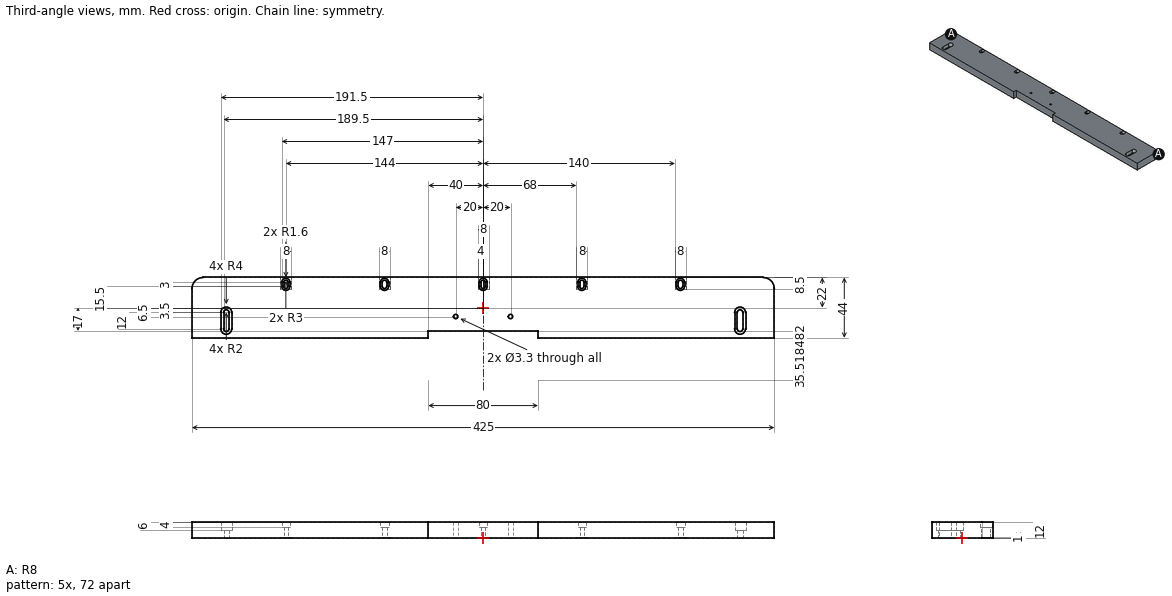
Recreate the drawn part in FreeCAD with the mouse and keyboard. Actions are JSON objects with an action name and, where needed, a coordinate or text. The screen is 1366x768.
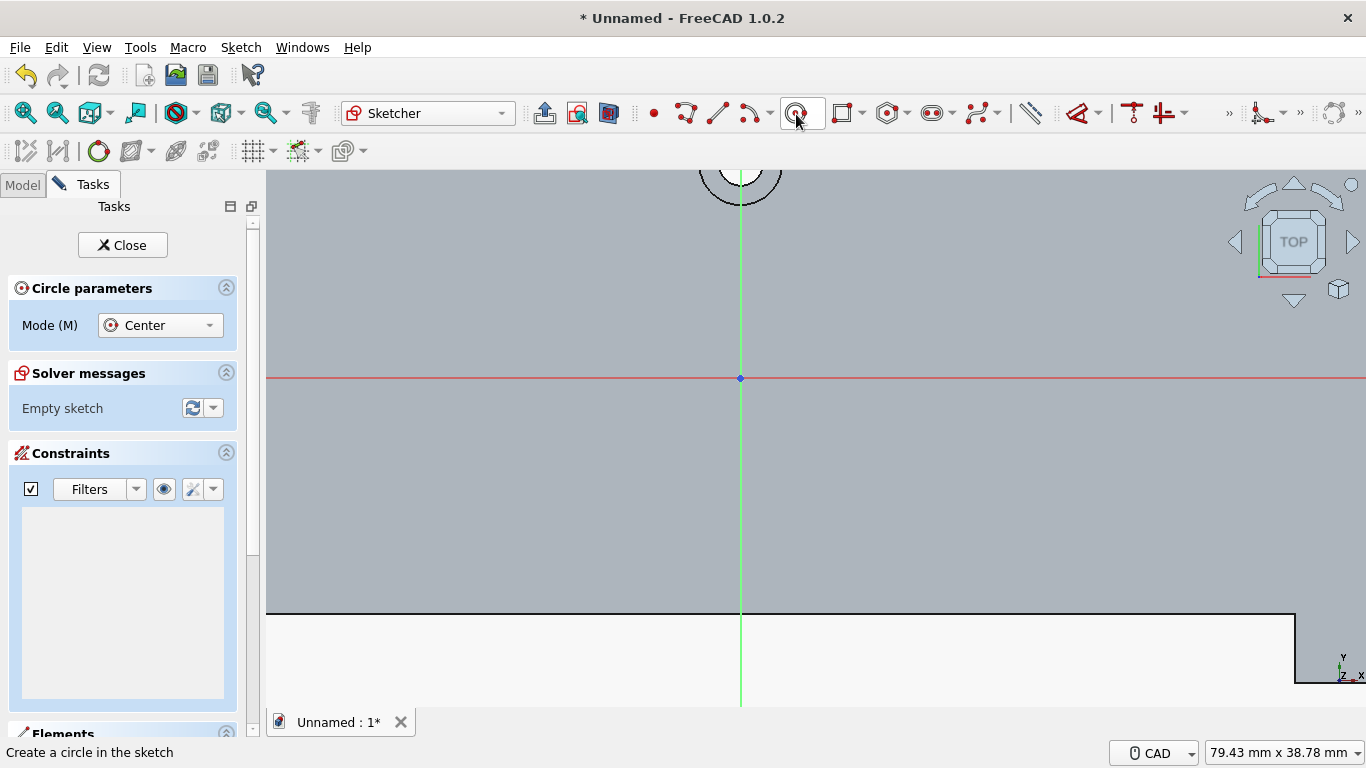
{"action": "left_click", "coordinate": [464, 468]}
{"action": "mouse_move", "coordinate": [480, 452]}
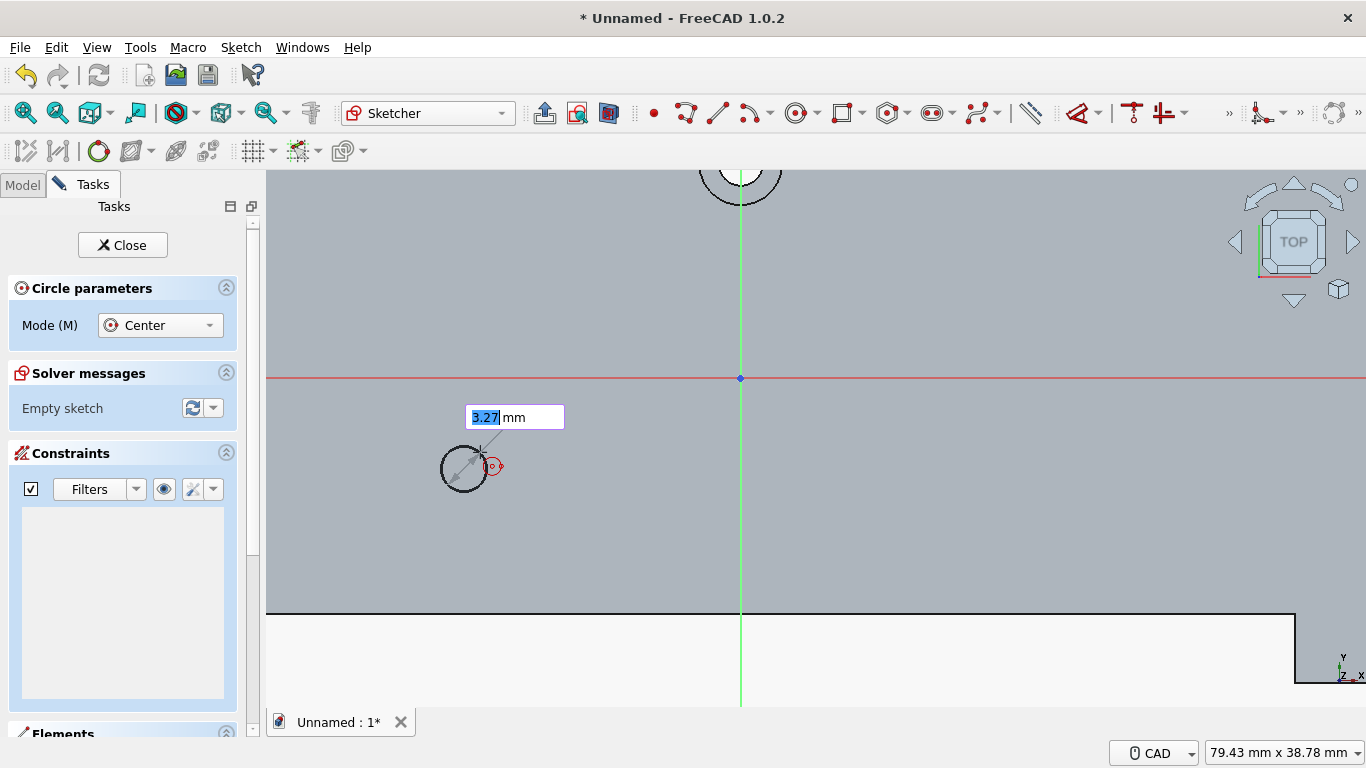
{"action": "type", "text": "3.3"}
{"action": "key", "text": "Return"}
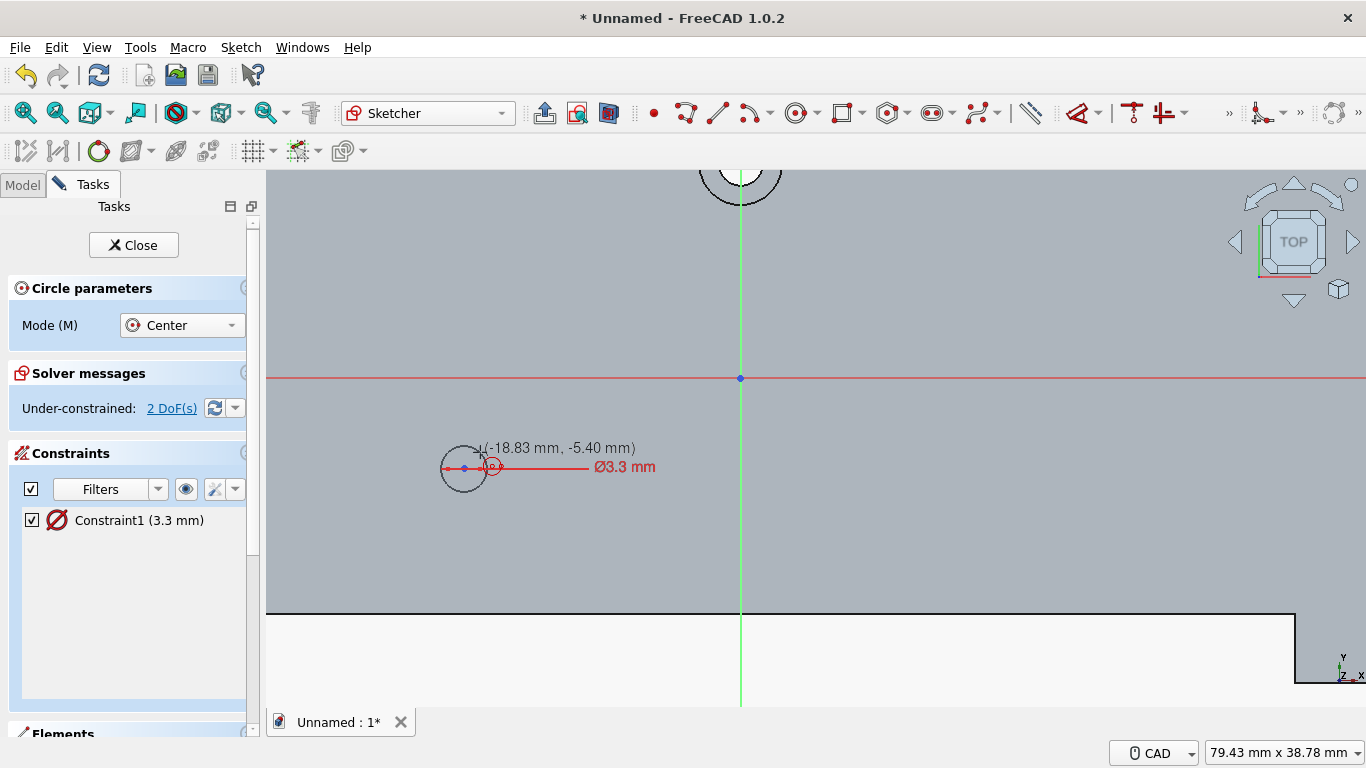
{"action": "left_click", "coordinate": [1018, 468]}
{"action": "mouse_move", "coordinate": [1034, 452]}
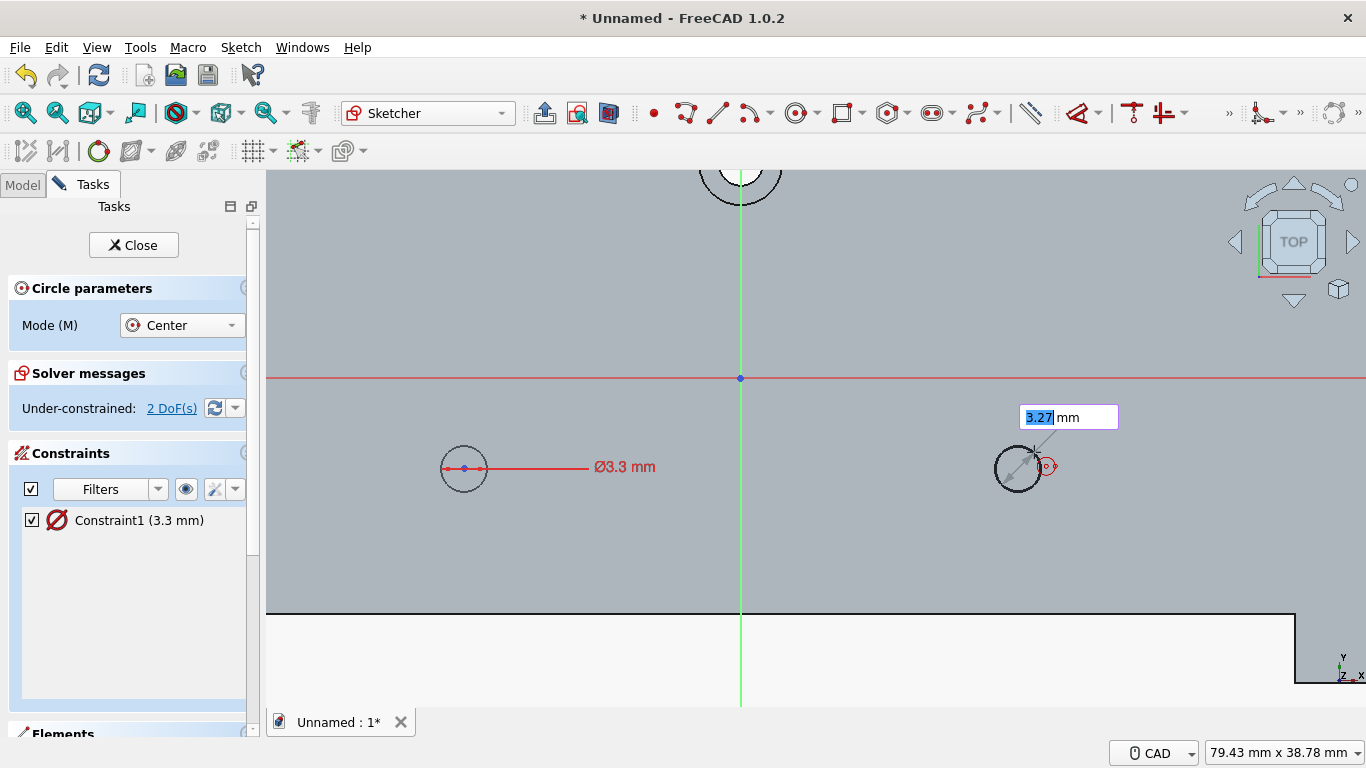
{"action": "type", "text": "3.3"}
{"action": "key", "text": "Return"}
{"action": "key", "text": "Escape"}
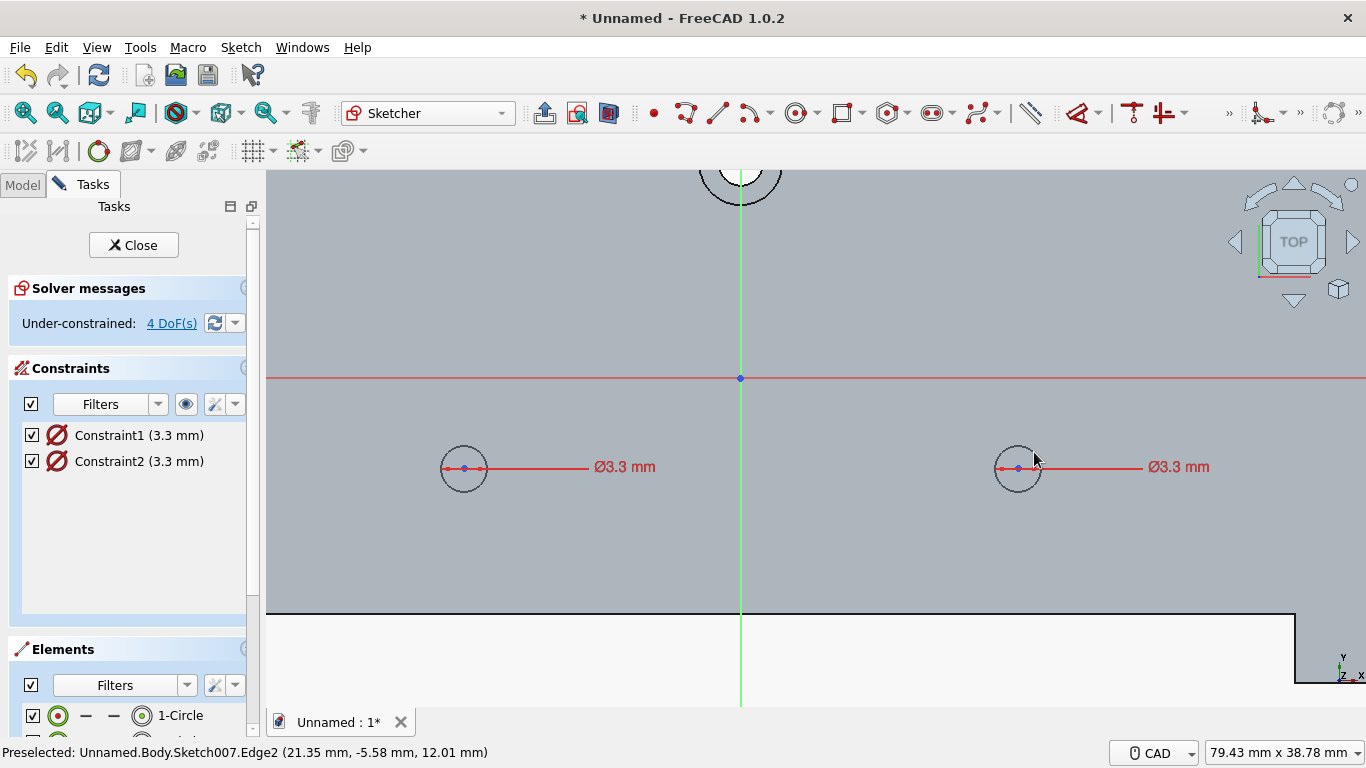
{"action": "left_click", "coordinate": [464, 469]}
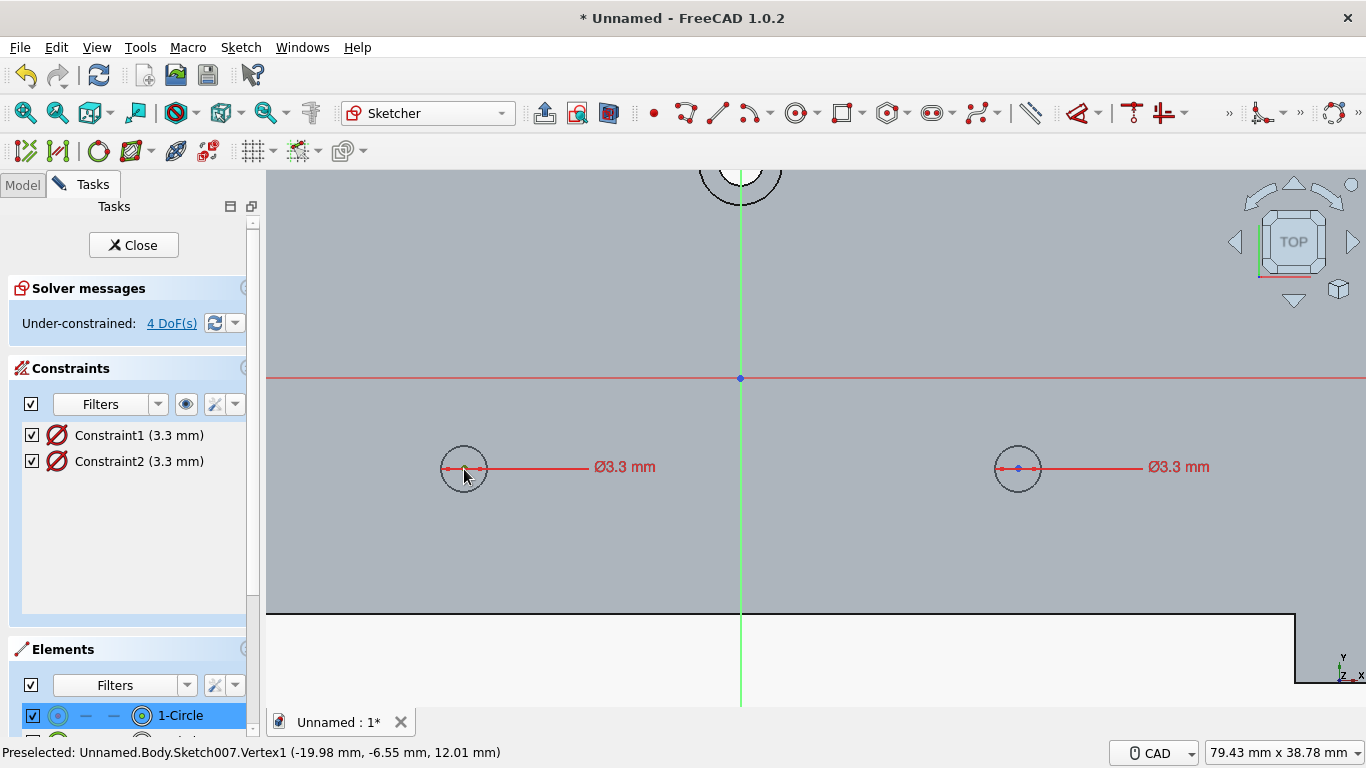
{"action": "left_click", "coordinate": [1018, 469]}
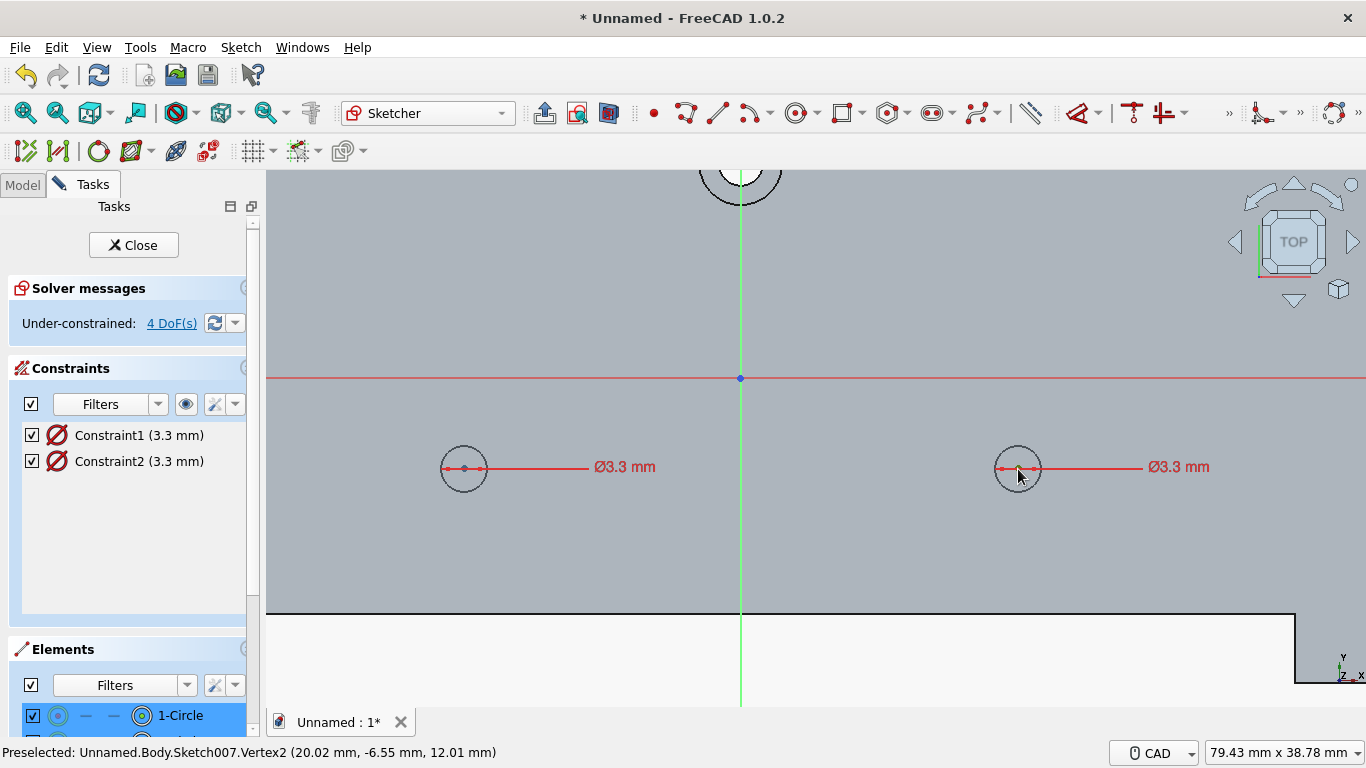
{"action": "key", "text": "h"}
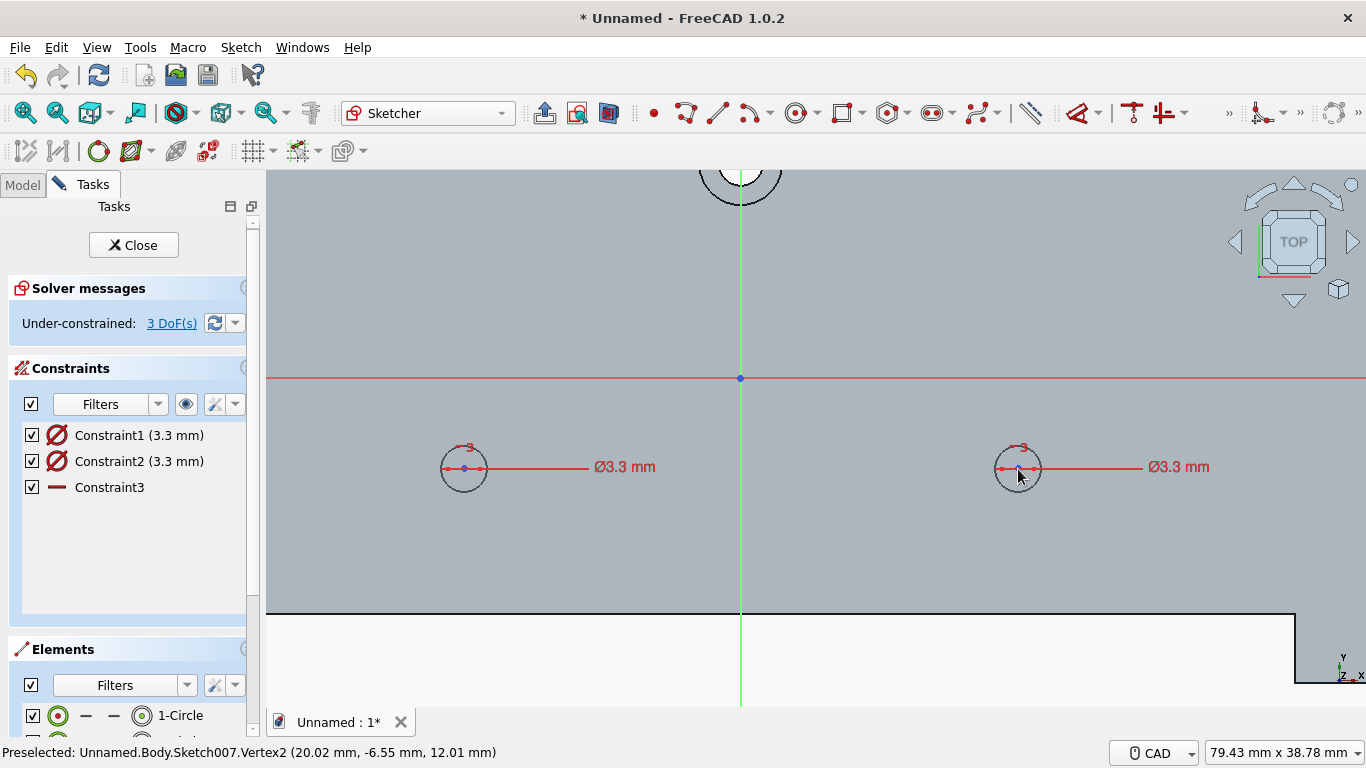
{"action": "left_click", "coordinate": [1078, 114]}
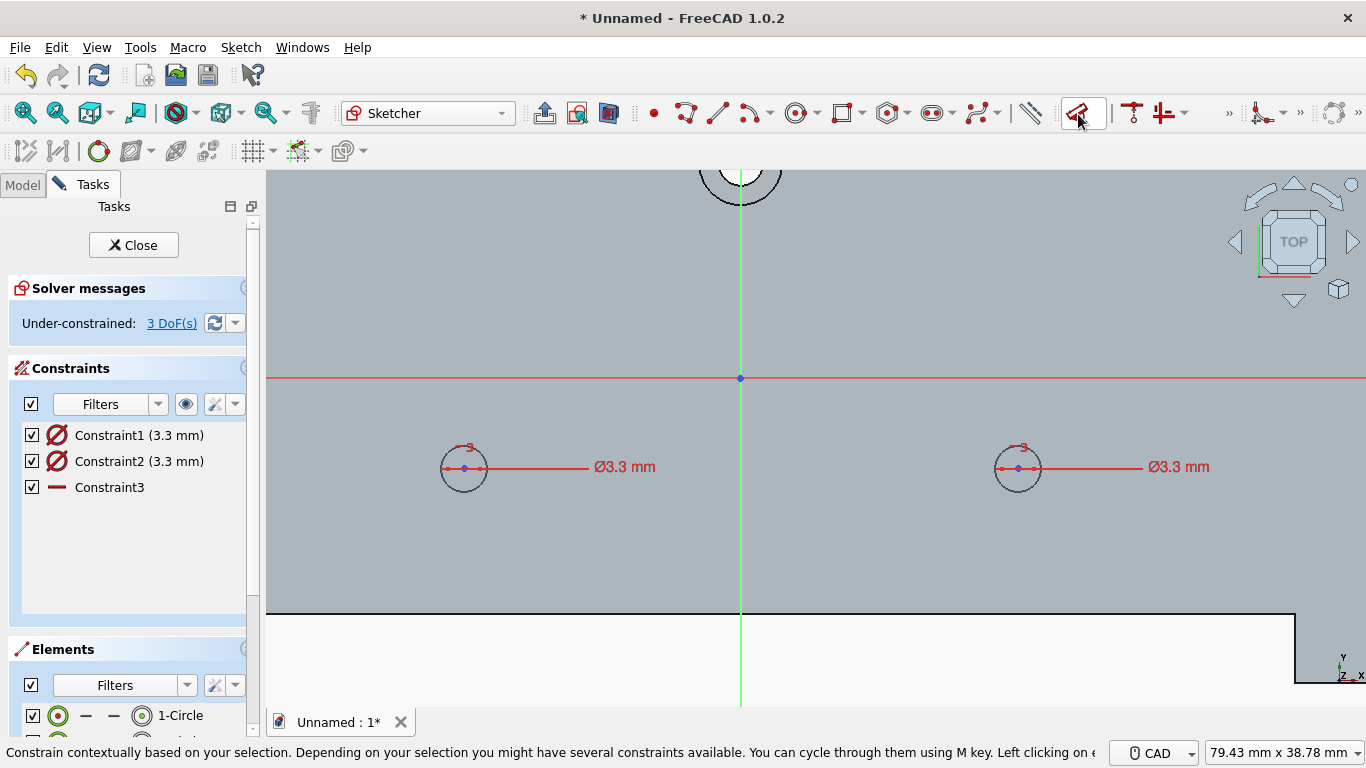
{"action": "left_click", "coordinate": [464, 469]}
{"action": "left_click", "coordinate": [602, 344]}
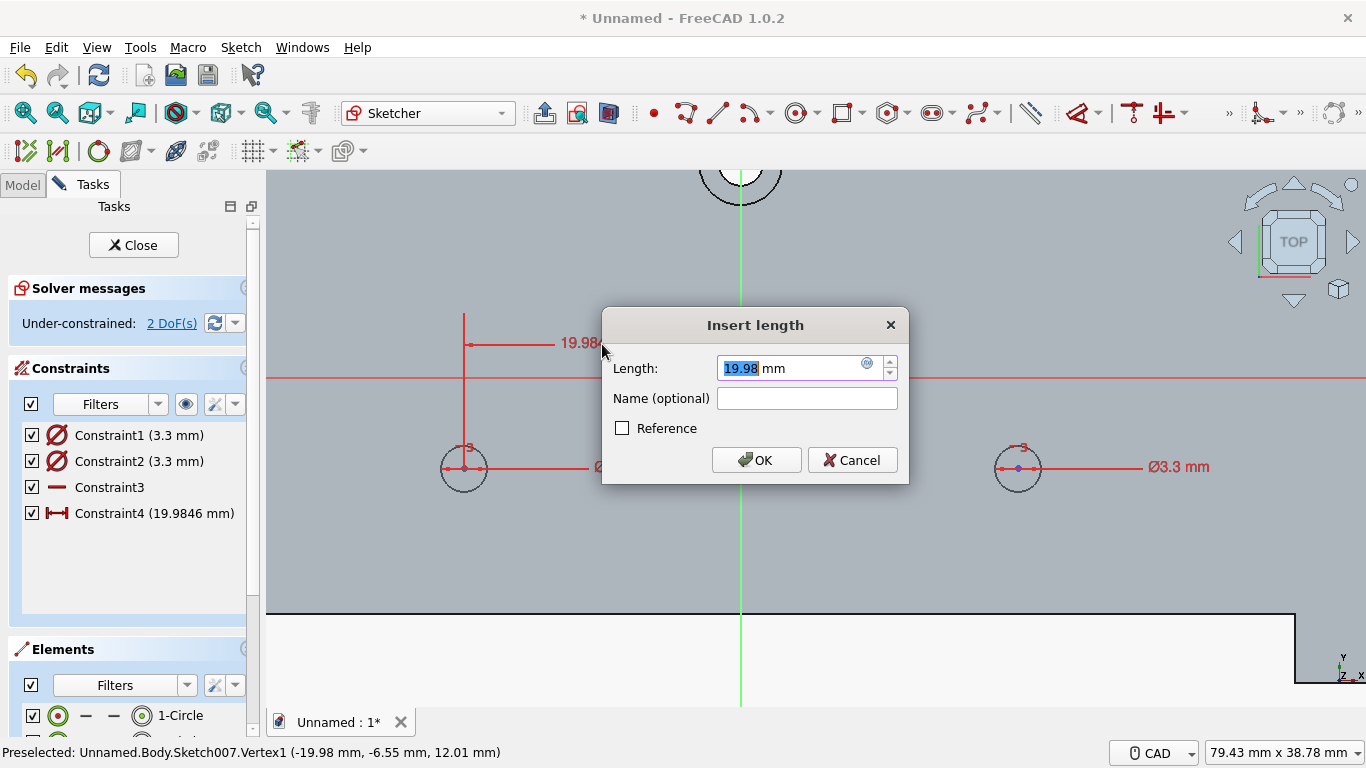
{"action": "type", "text": "20"}
{"action": "key", "text": "Return"}